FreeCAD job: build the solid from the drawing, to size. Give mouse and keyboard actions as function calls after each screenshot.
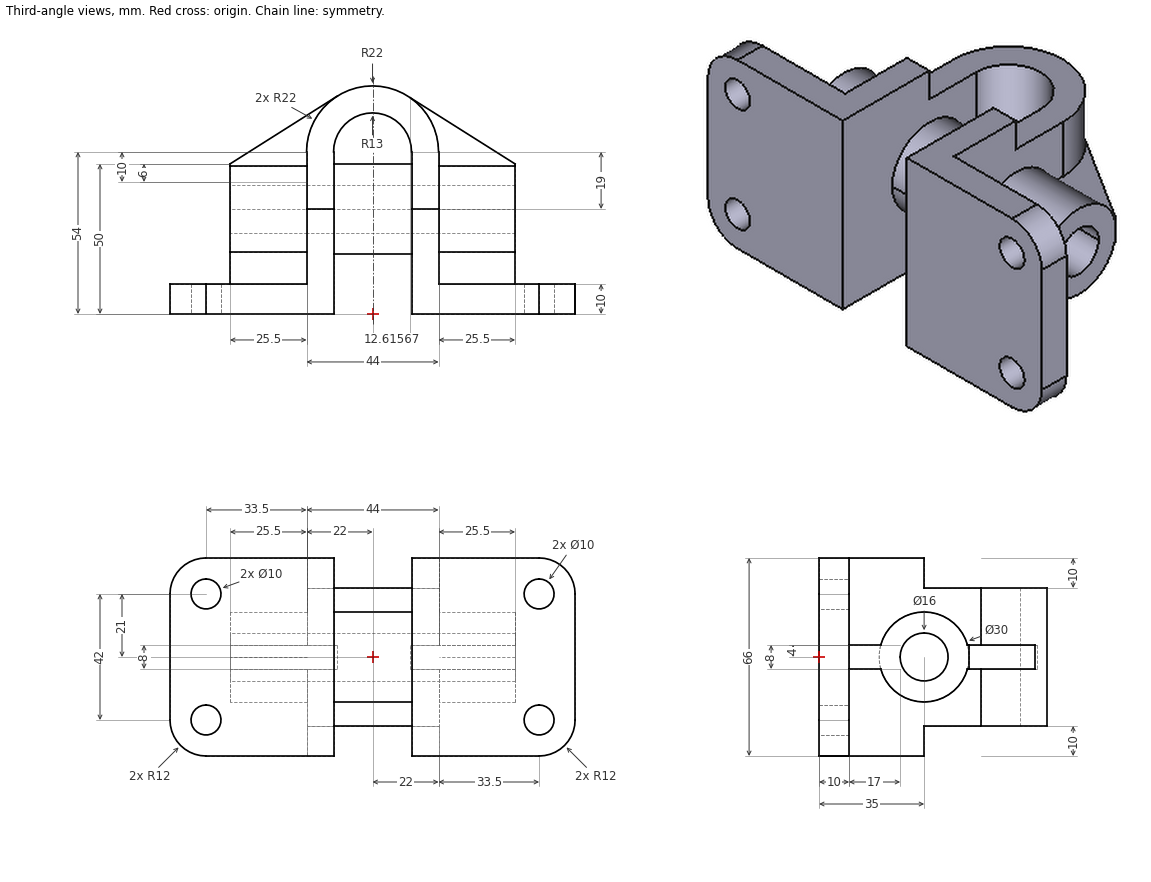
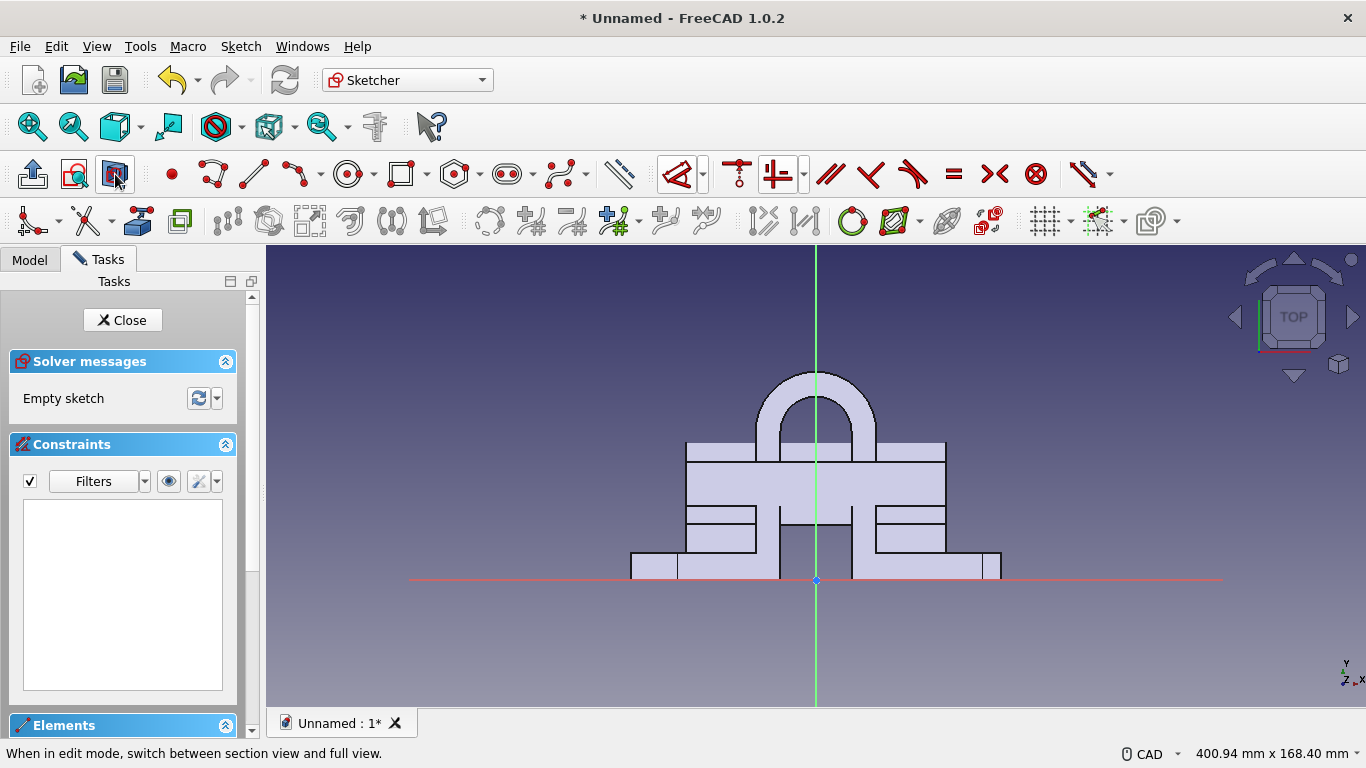
scroll(955, 490, up, 2)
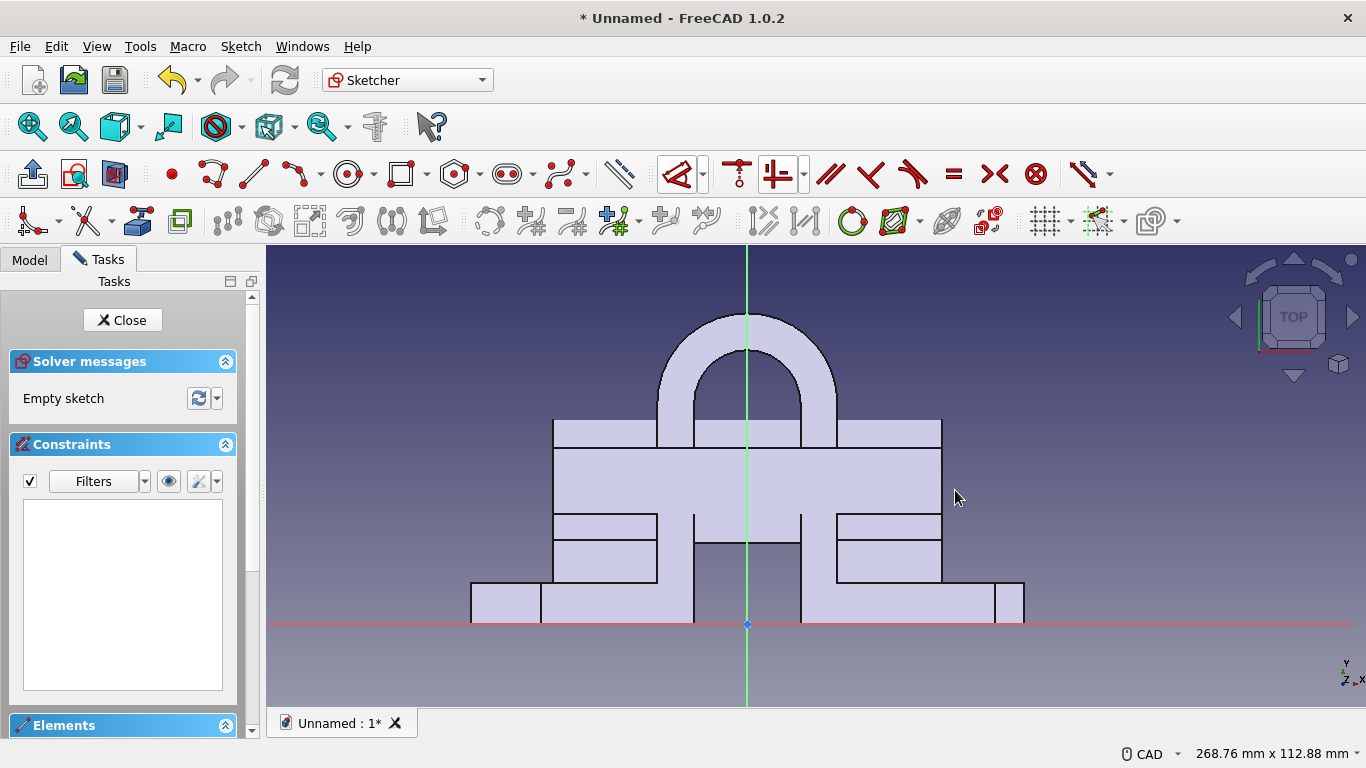
click(213, 174)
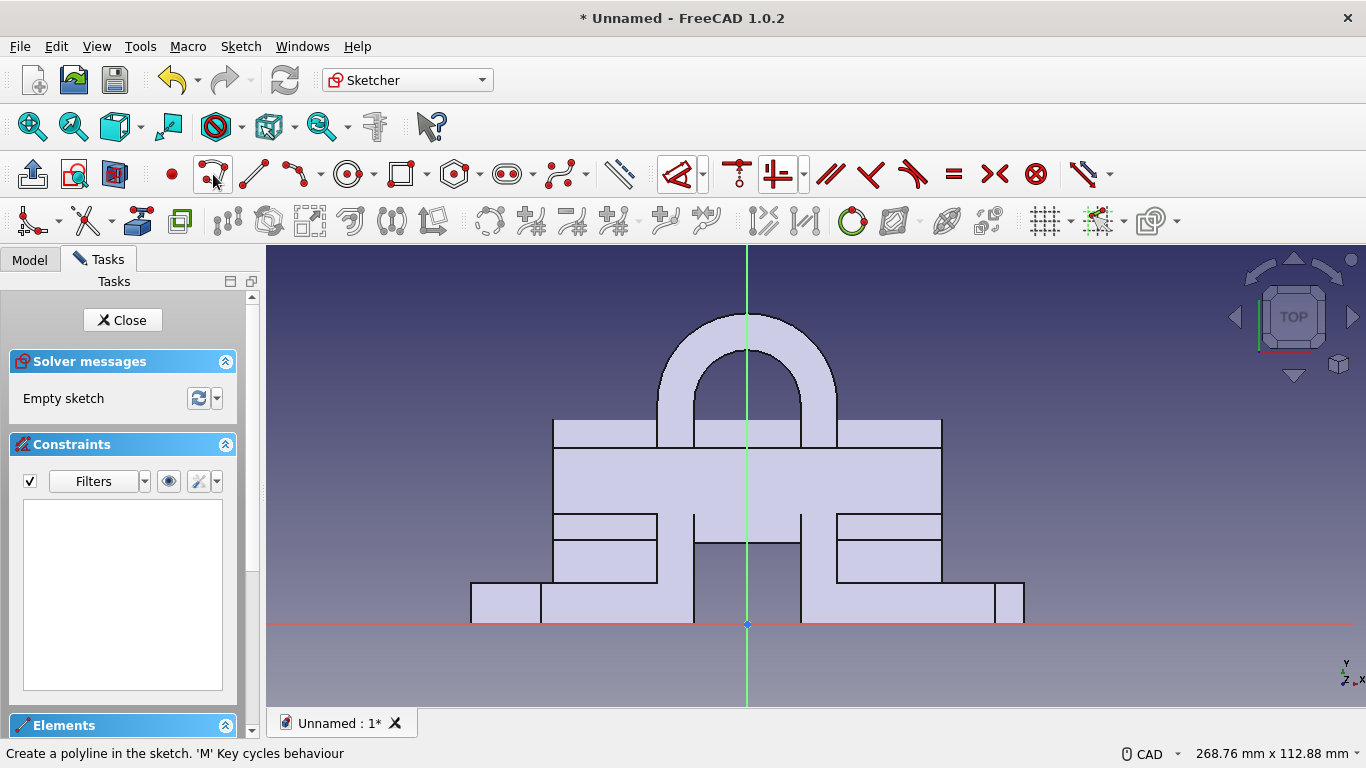
click(699, 327)
click(553, 420)
click(553, 444)
click(657, 444)
click(657, 403)
right_click(657, 403)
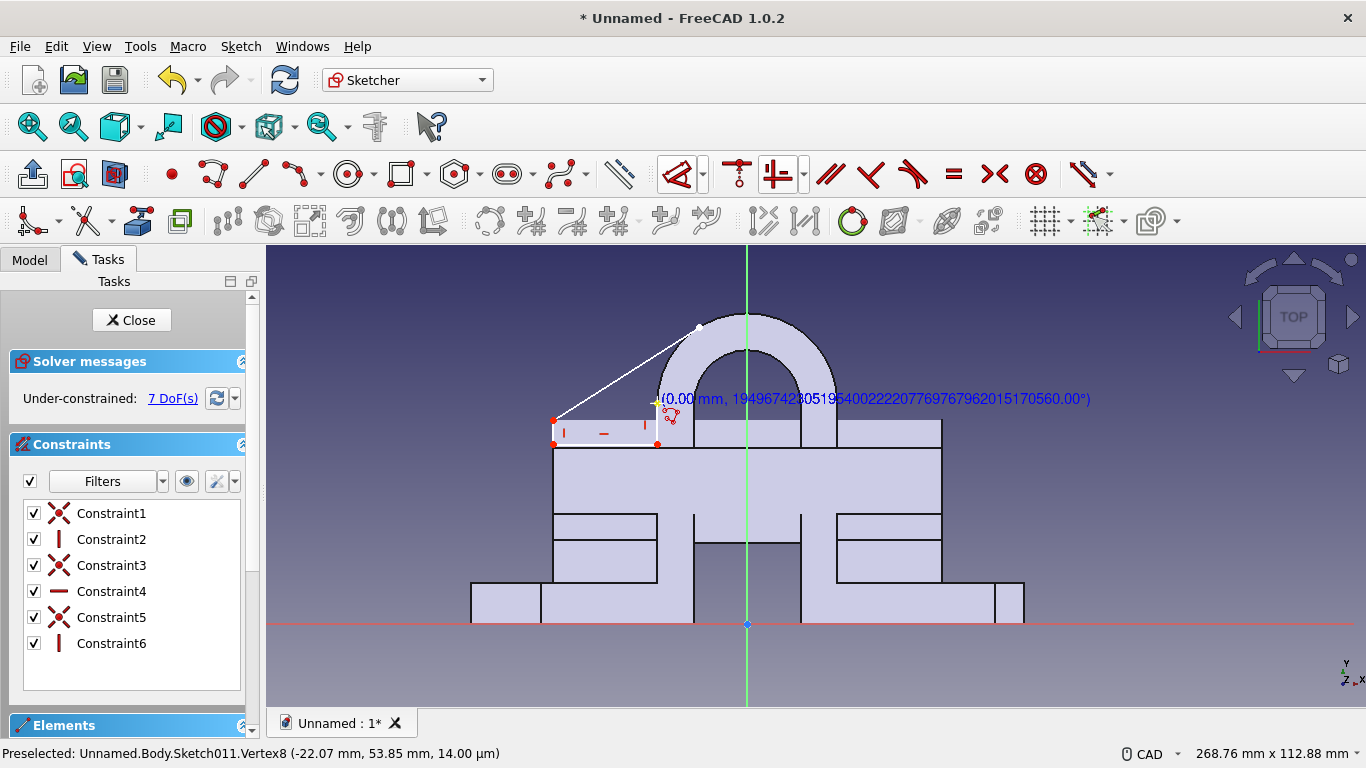
click(294, 174)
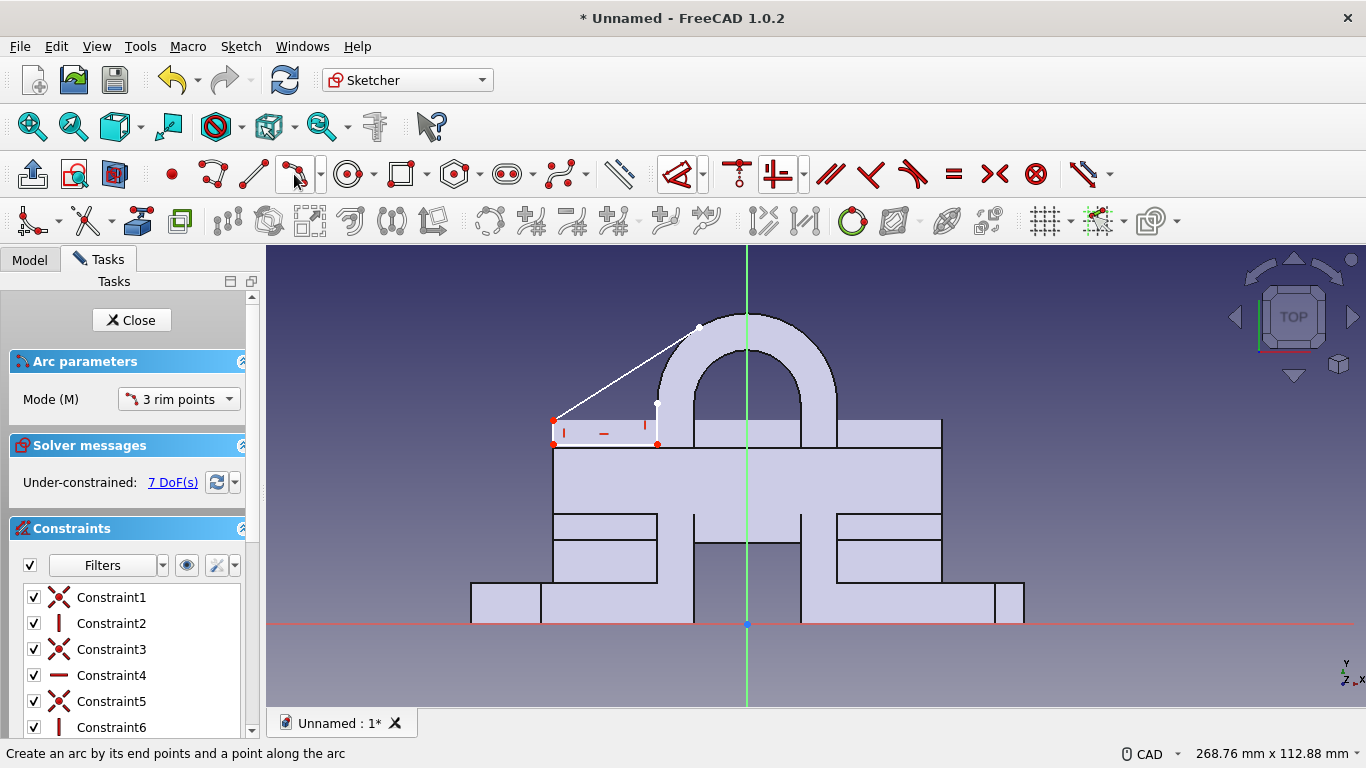
click(657, 404)
click(699, 328)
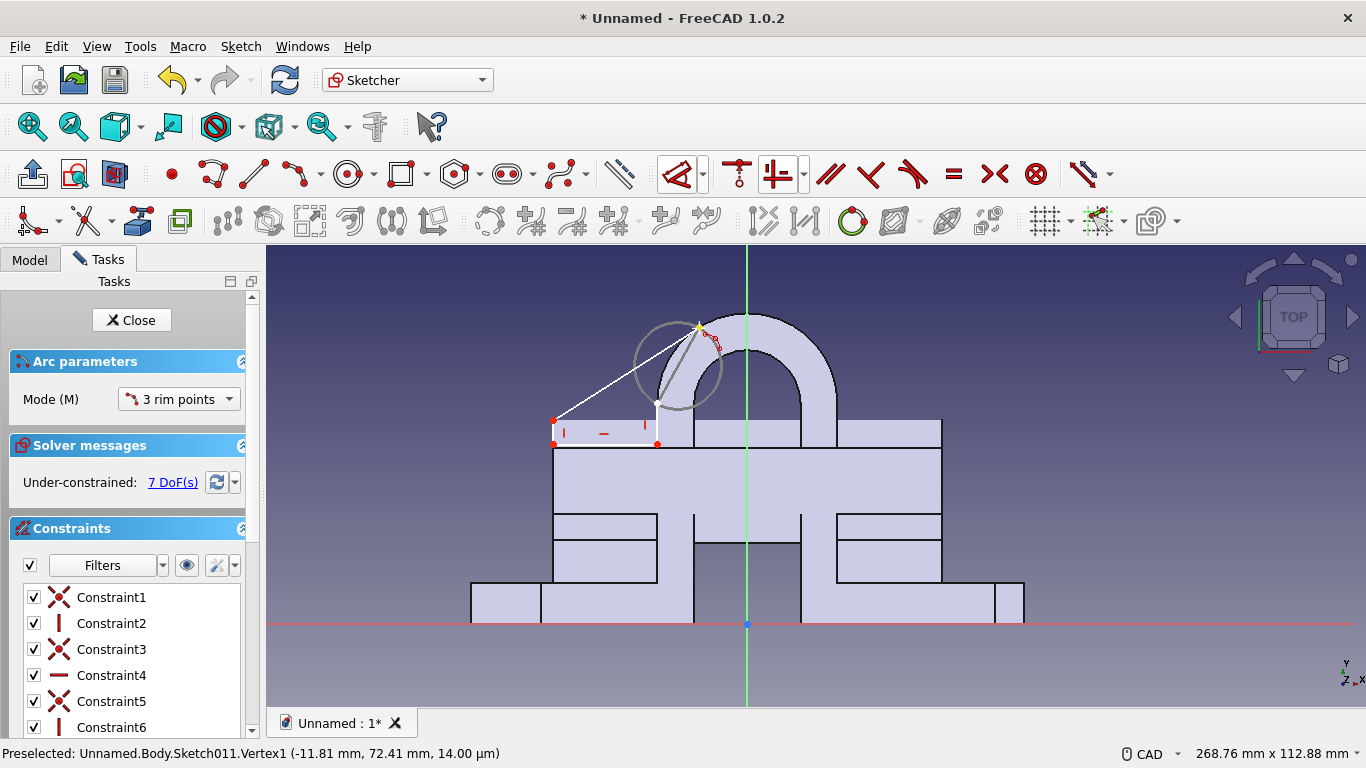
scroll(668, 360, up, 2)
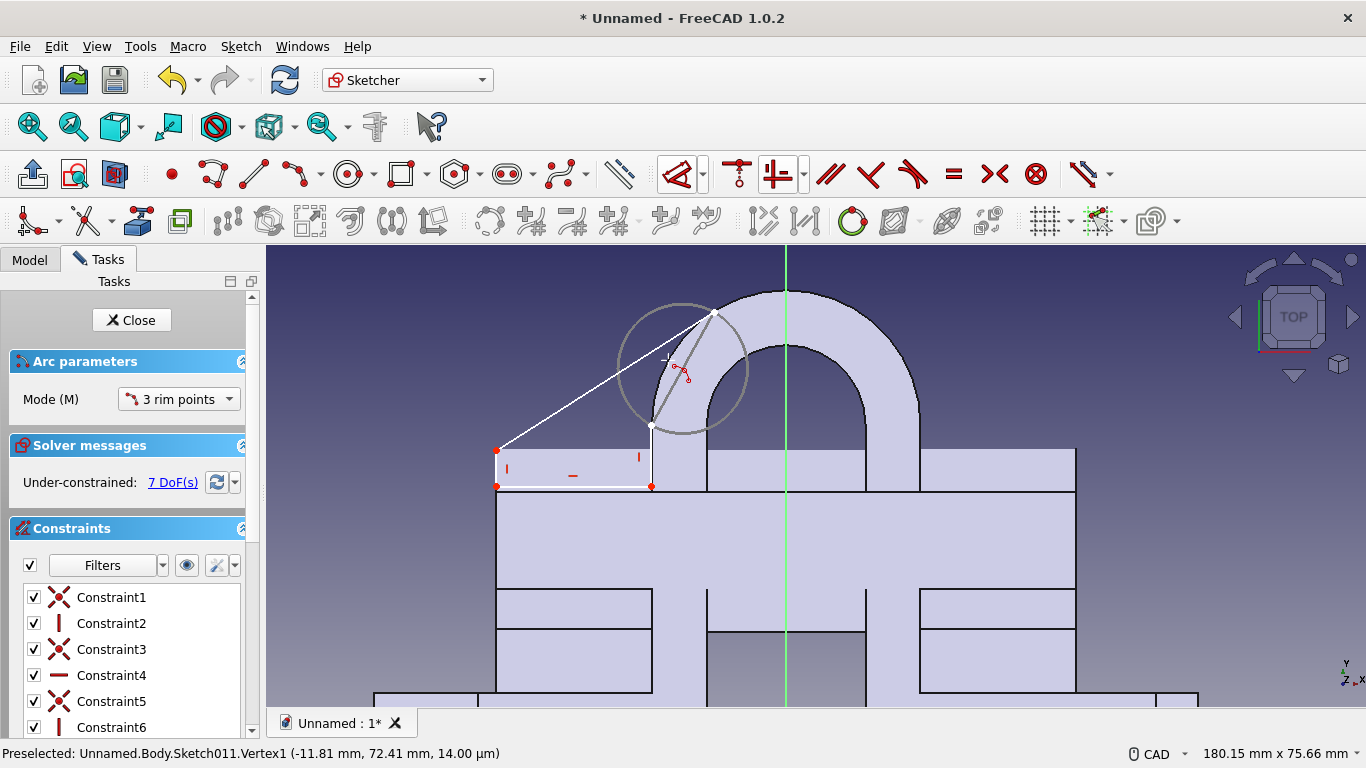
click(669, 360)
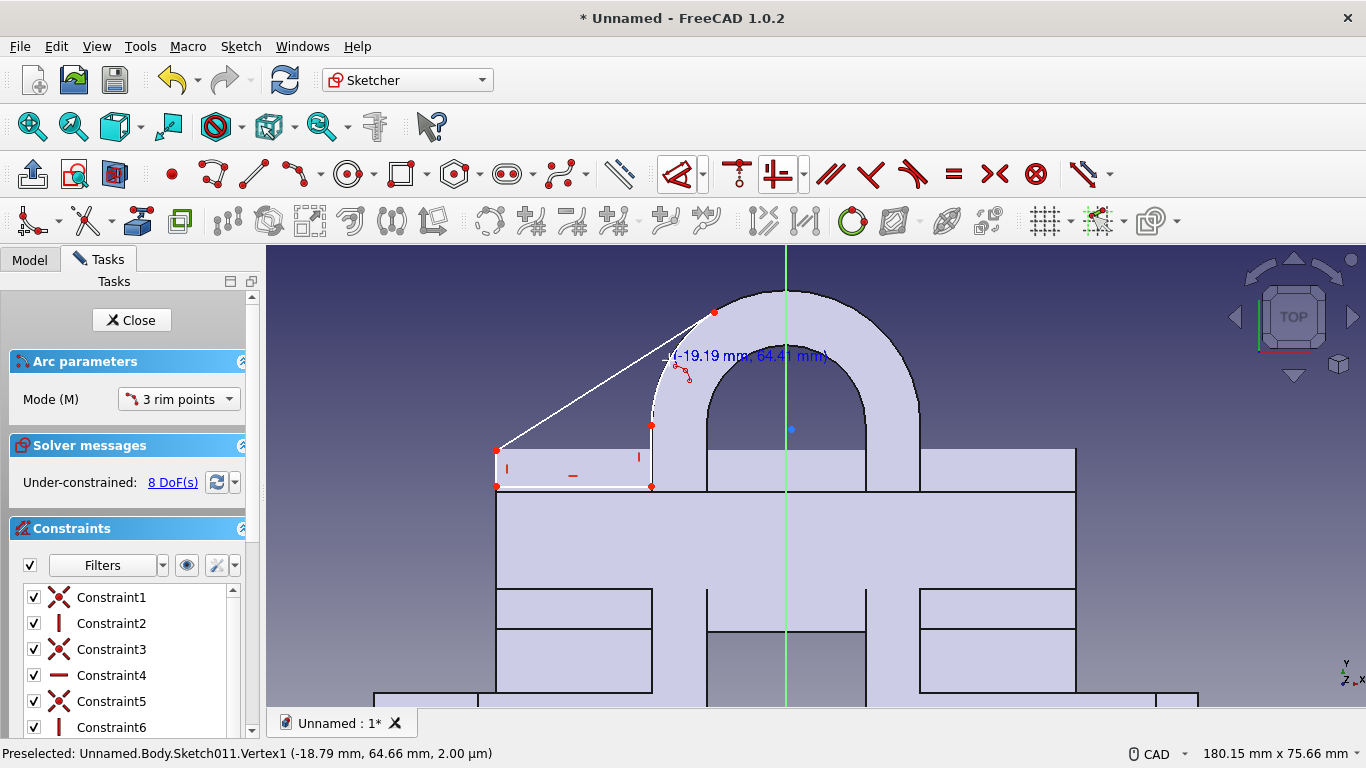
click(213, 174)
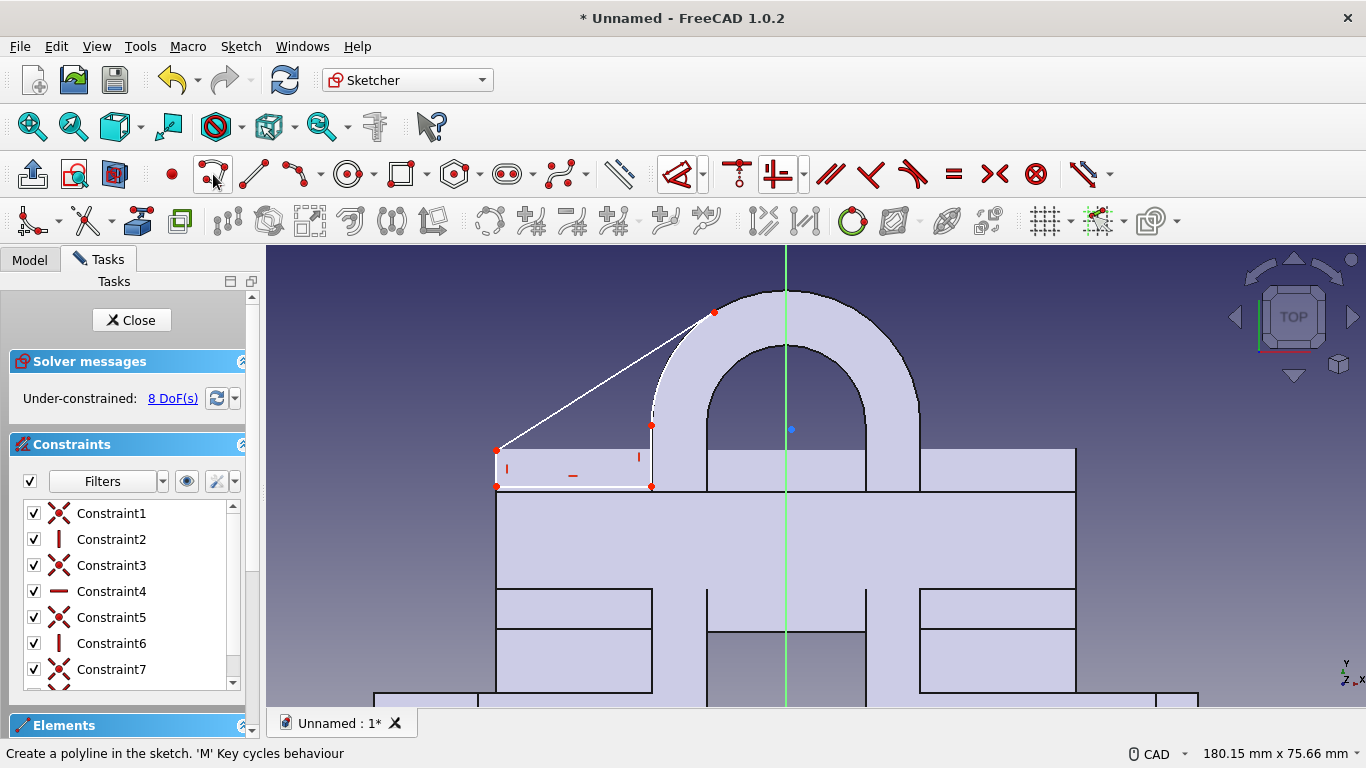
click(920, 425)
click(920, 486)
click(1076, 486)
click(1076, 449)
click(863, 315)
right_click(863, 315)